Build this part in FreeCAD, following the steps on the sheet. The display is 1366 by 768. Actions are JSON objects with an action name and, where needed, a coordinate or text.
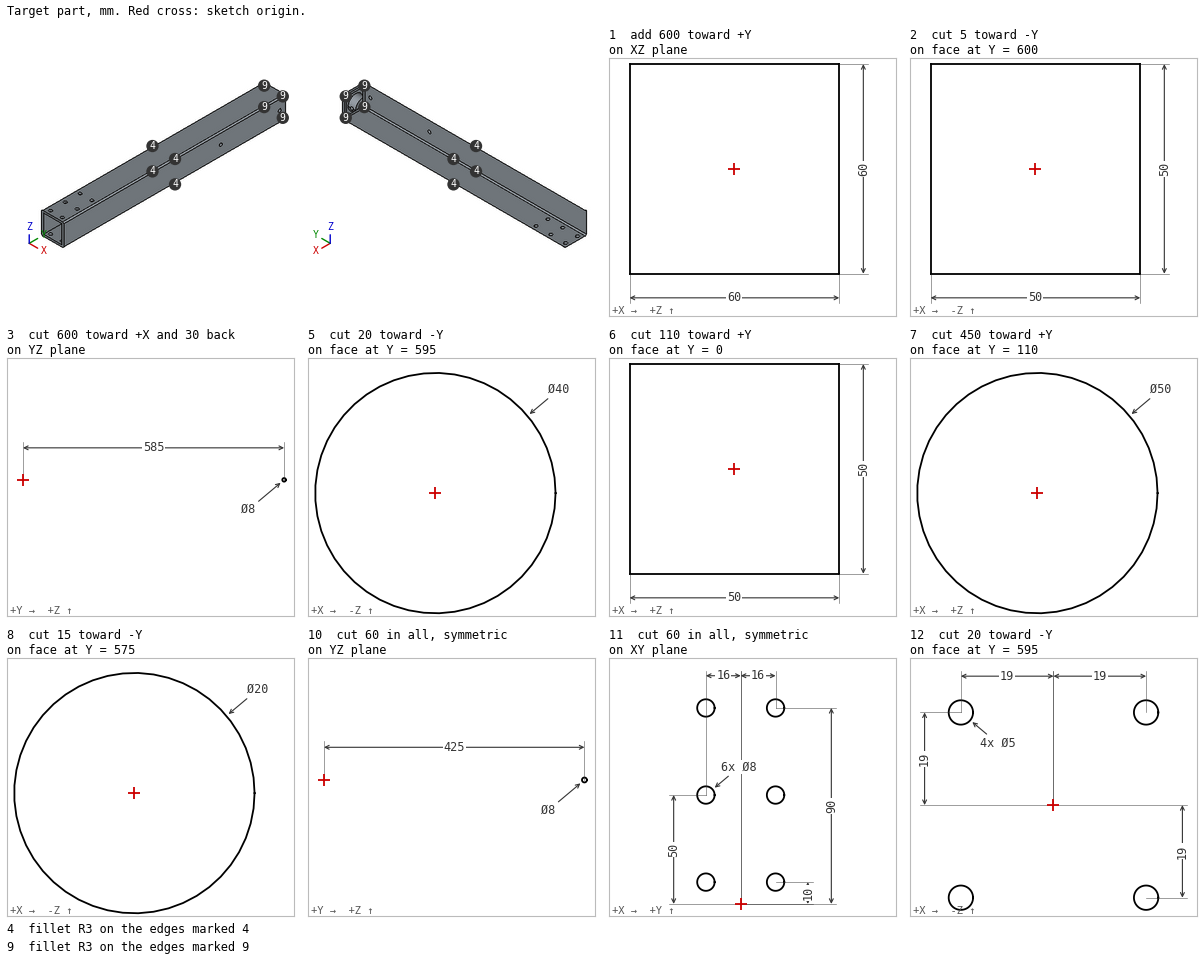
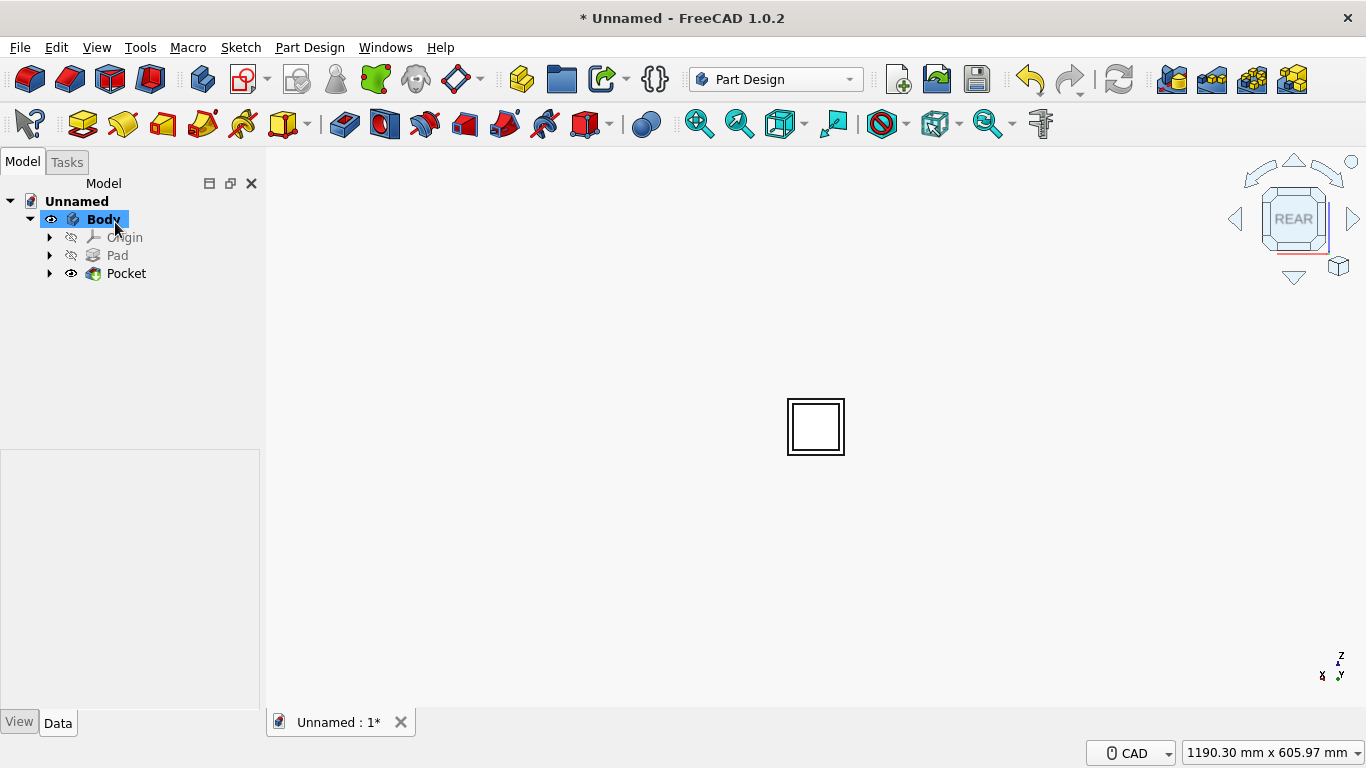
{"action": "left_click", "coordinate": [244, 80]}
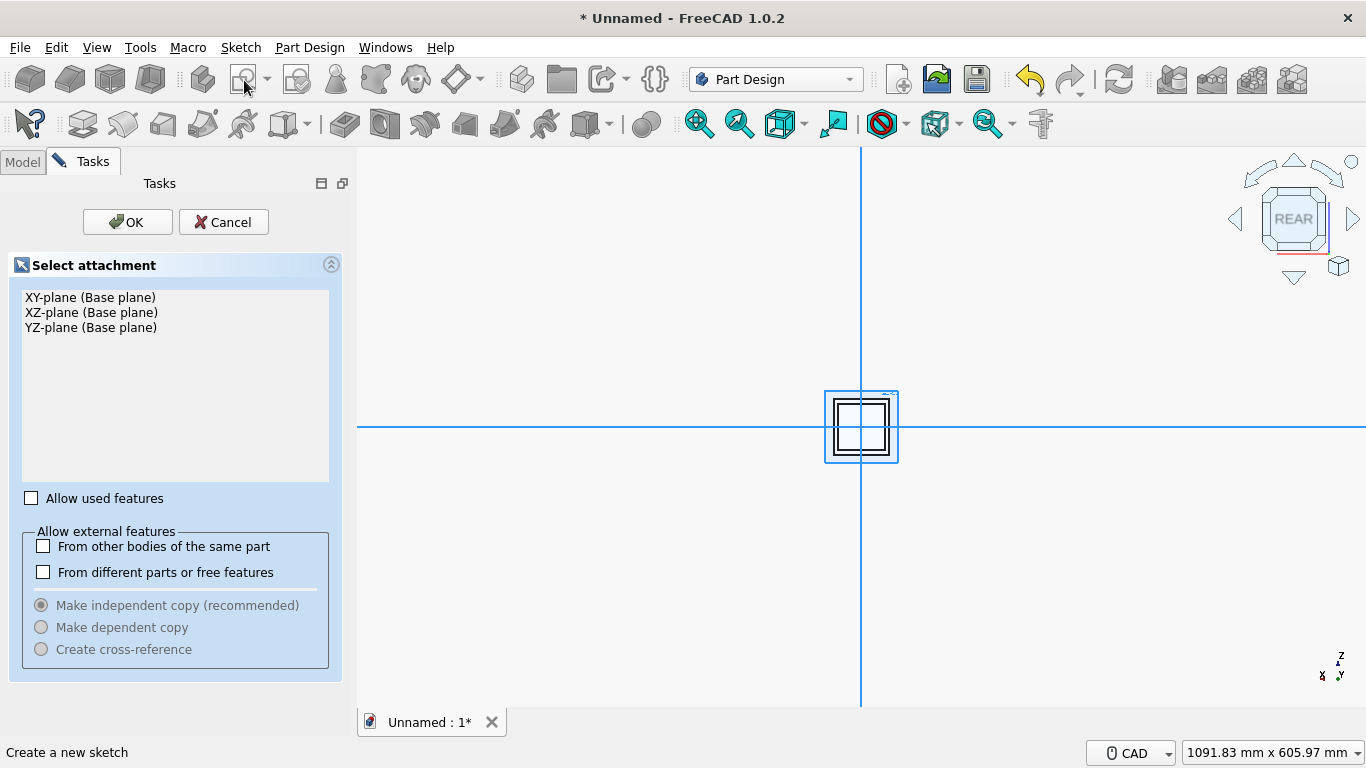
{"action": "left_click", "coordinate": [82, 328]}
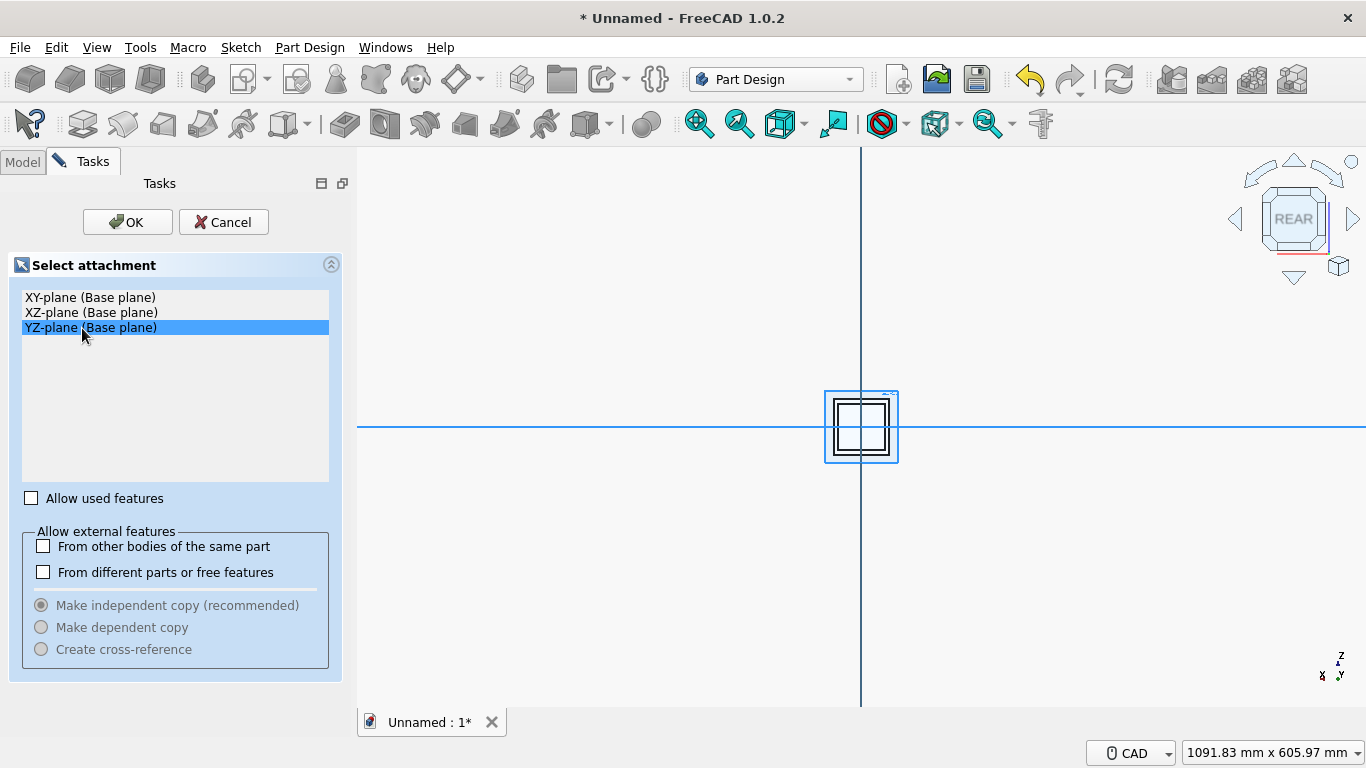
{"action": "left_click", "coordinate": [128, 222]}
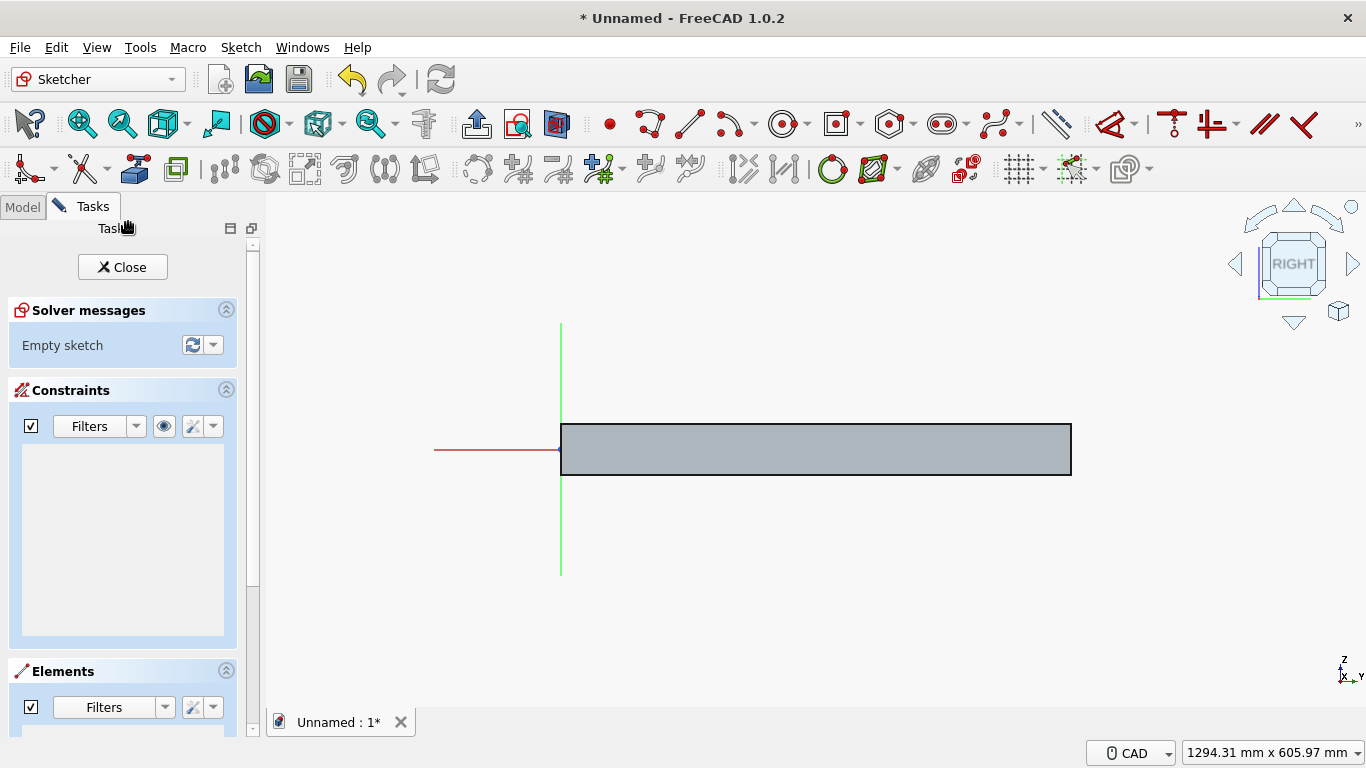
{"action": "key", "text": "q s"}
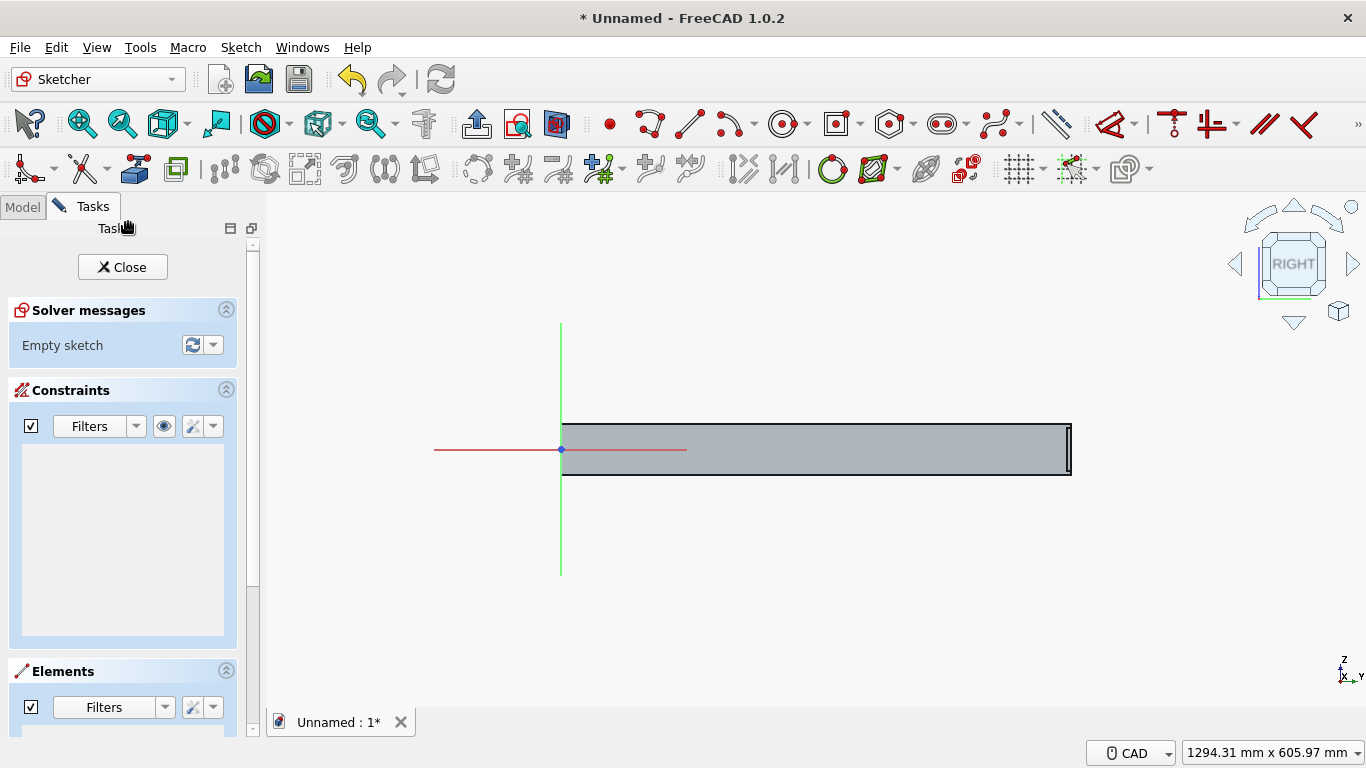
{"action": "scroll", "coordinate": [1074, 450], "scroll_direction": "up", "scroll_amount": 15}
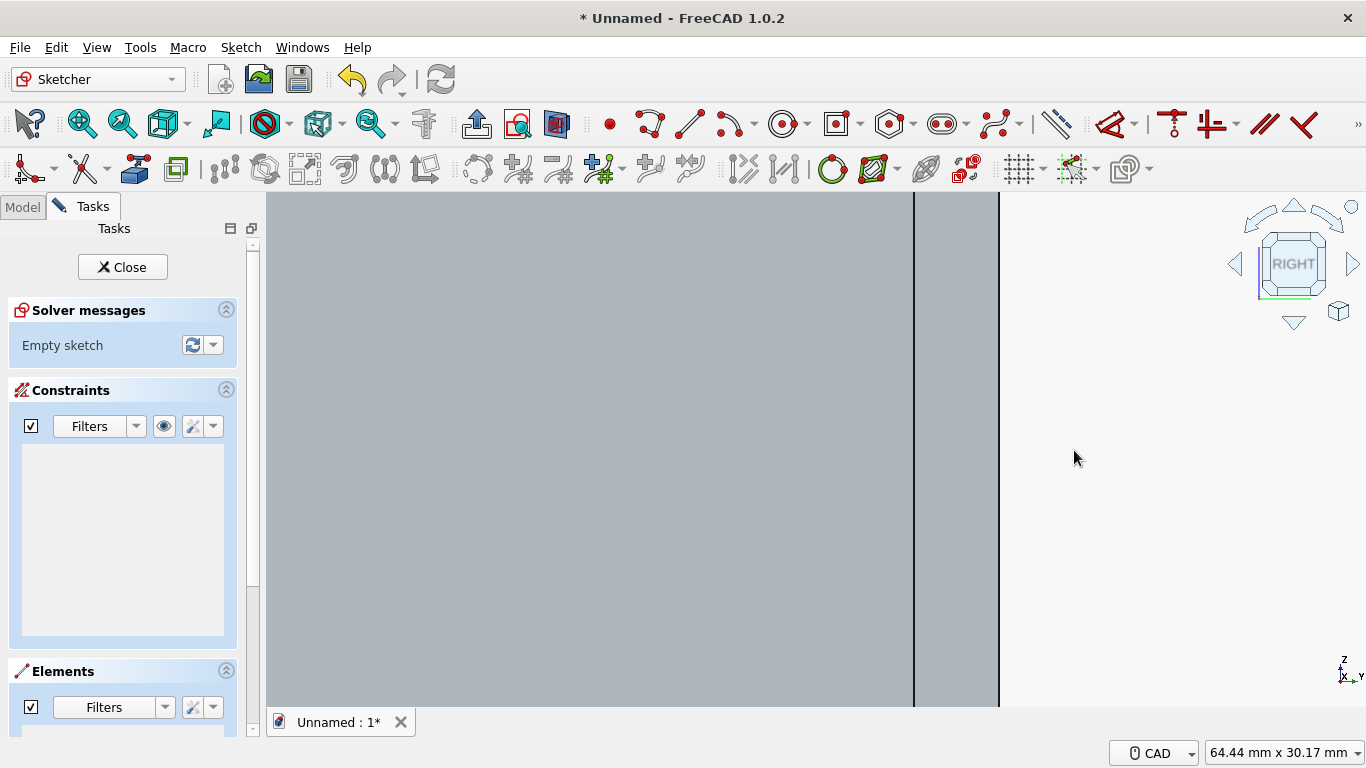
{"action": "scroll", "coordinate": [739, 415], "scroll_direction": "up", "scroll_amount": 4}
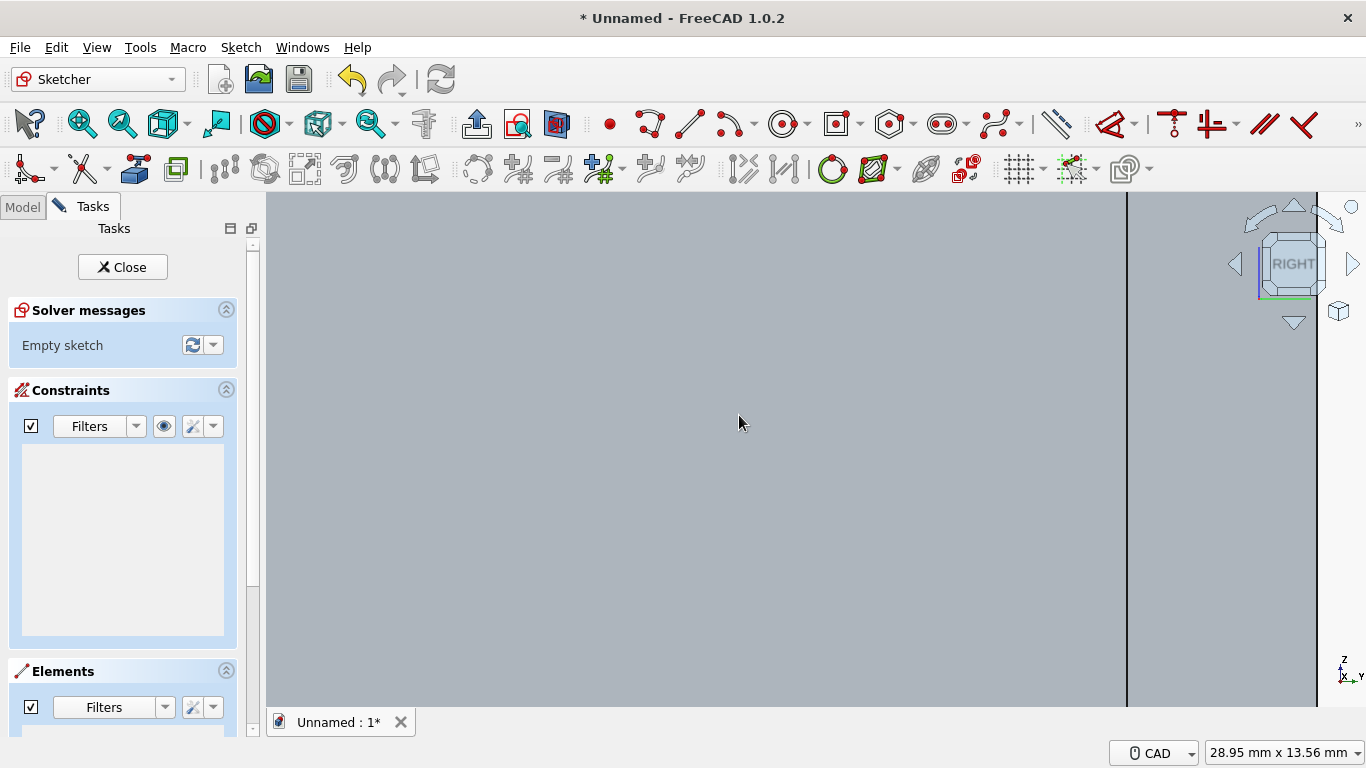
{"action": "left_click", "coordinate": [784, 124]}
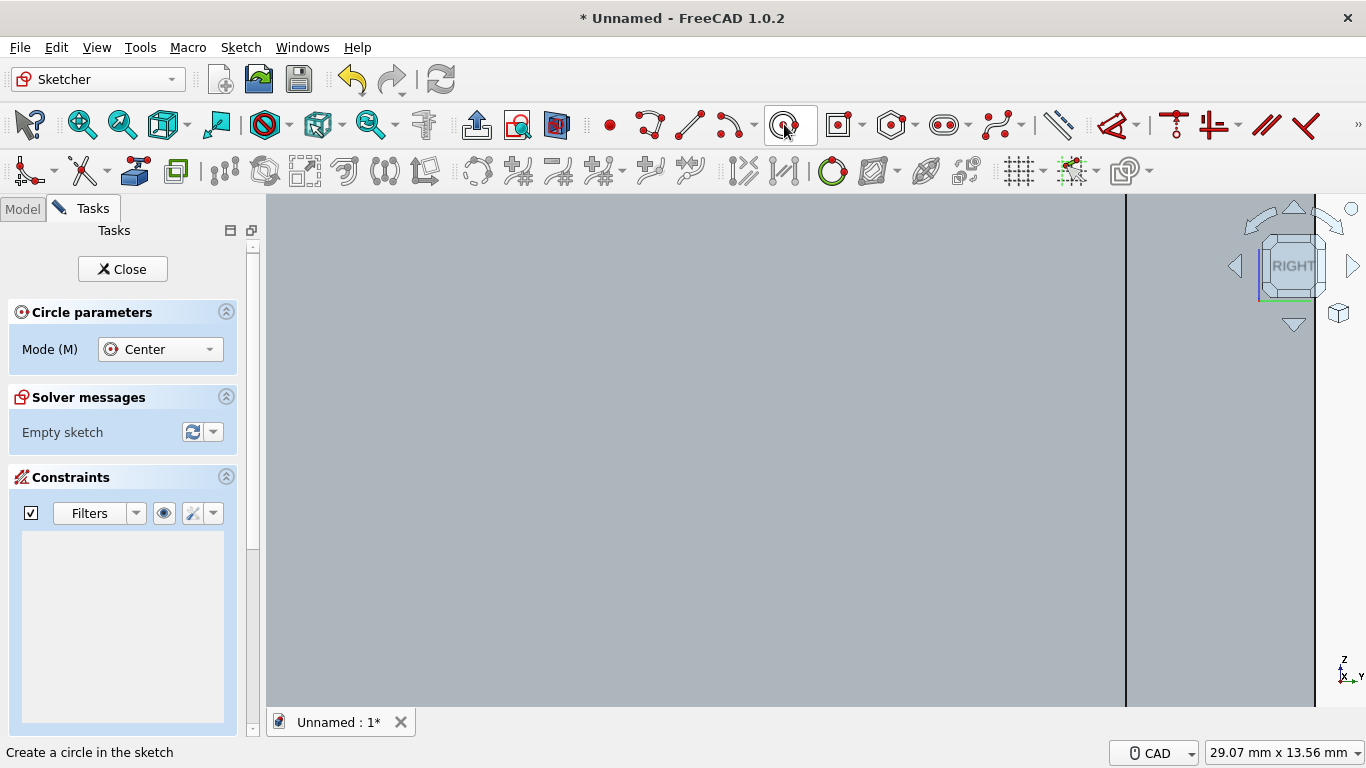
{"action": "left_click", "coordinate": [747, 450]}
{"action": "mouse_move", "coordinate": [854, 343]}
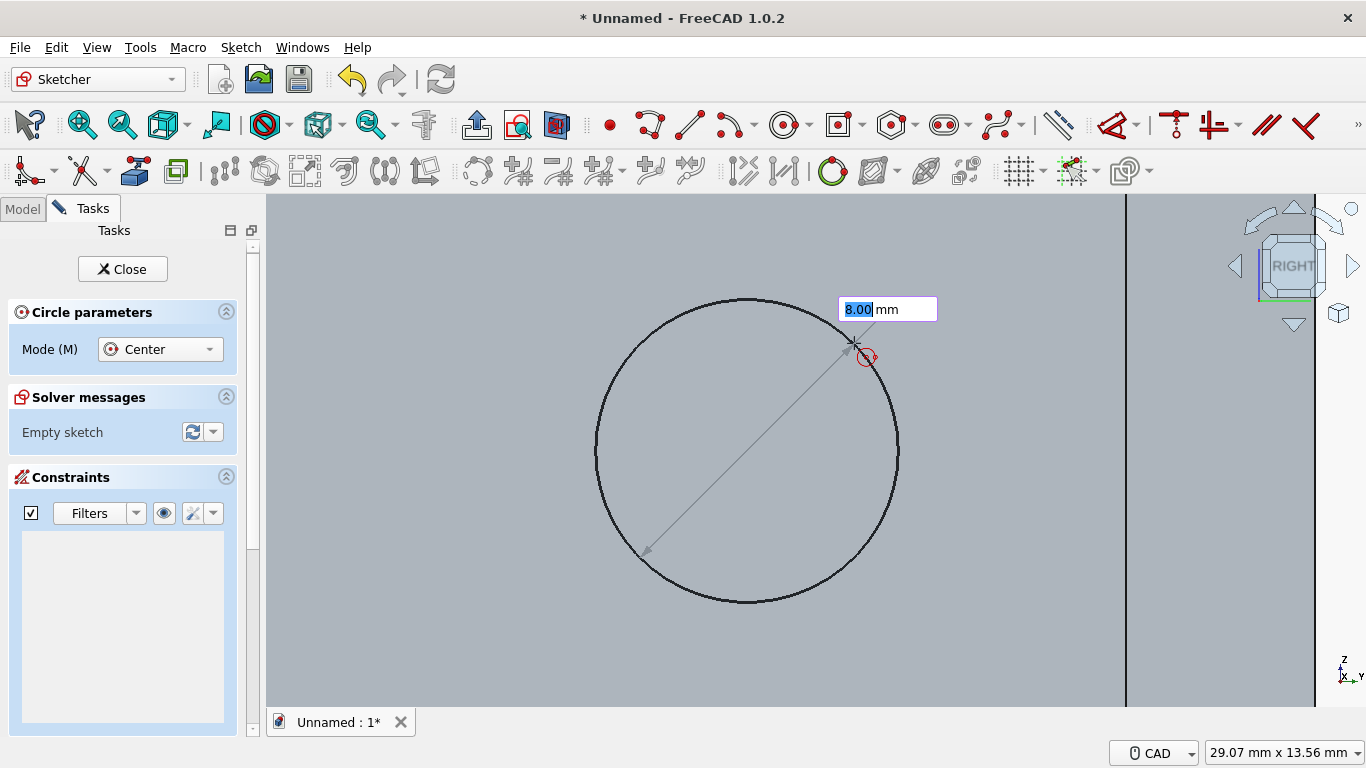
{"action": "type", "text": "8"}
{"action": "key", "text": "Return"}
{"action": "key", "text": "Escape"}